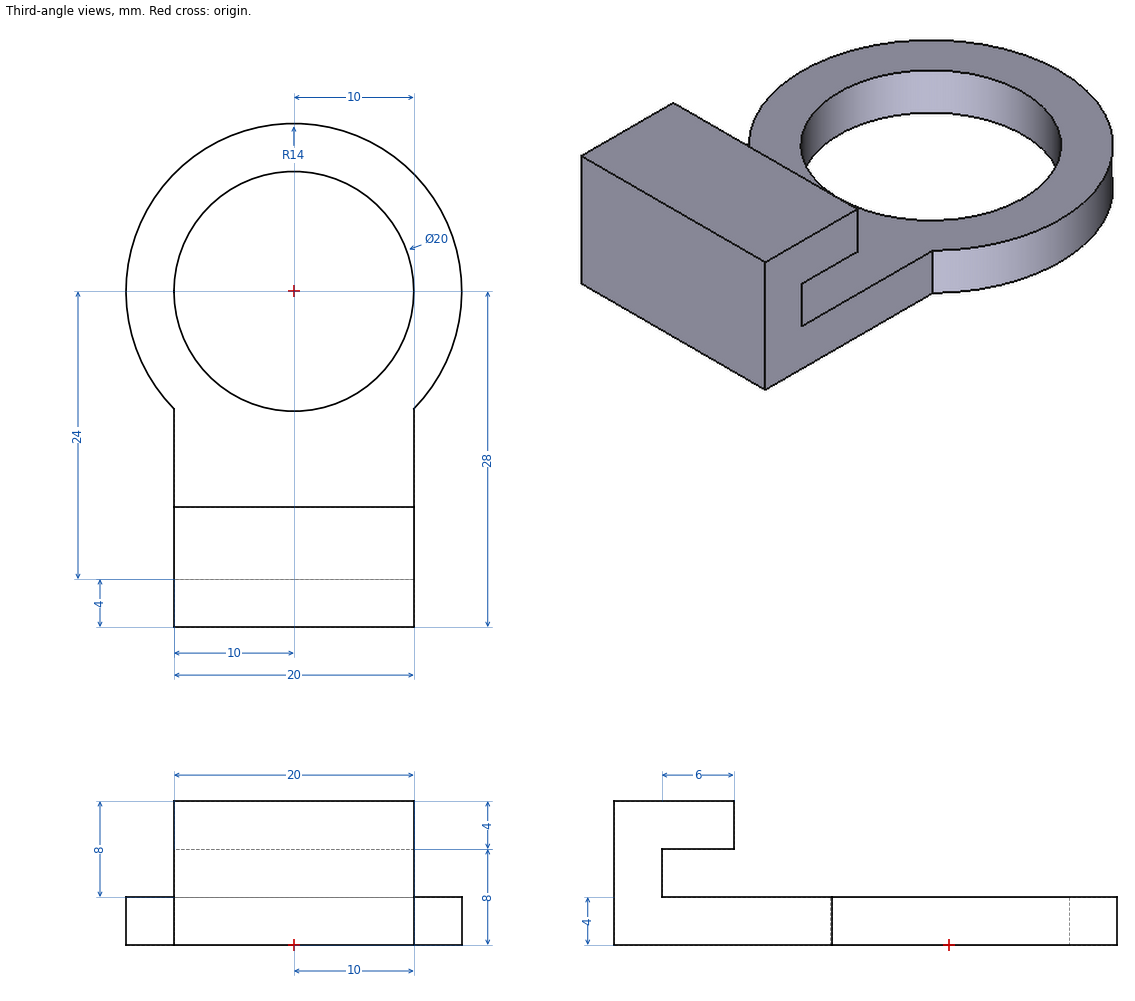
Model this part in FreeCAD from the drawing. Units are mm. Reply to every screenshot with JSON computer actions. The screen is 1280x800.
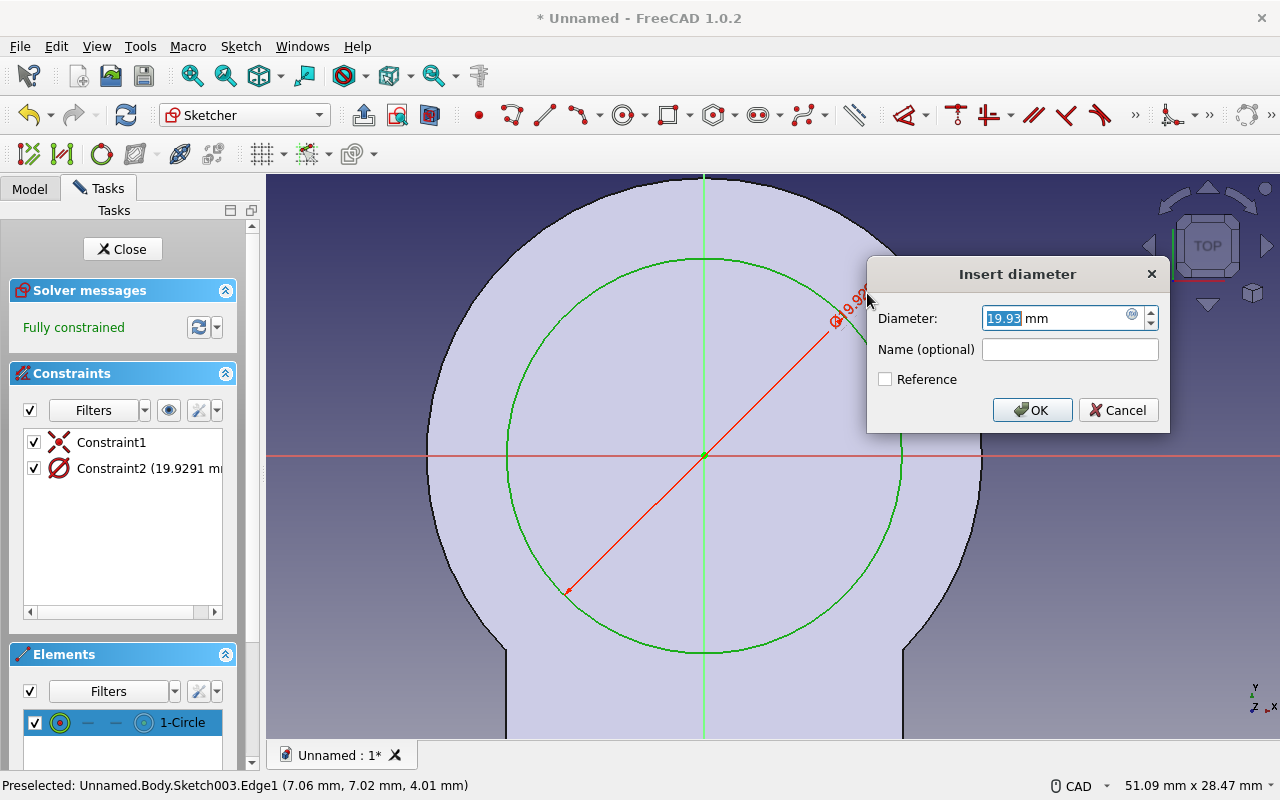
{"action": "type", "text": "20"}
{"action": "key", "text": "Return"}
{"action": "key", "text": "Escape"}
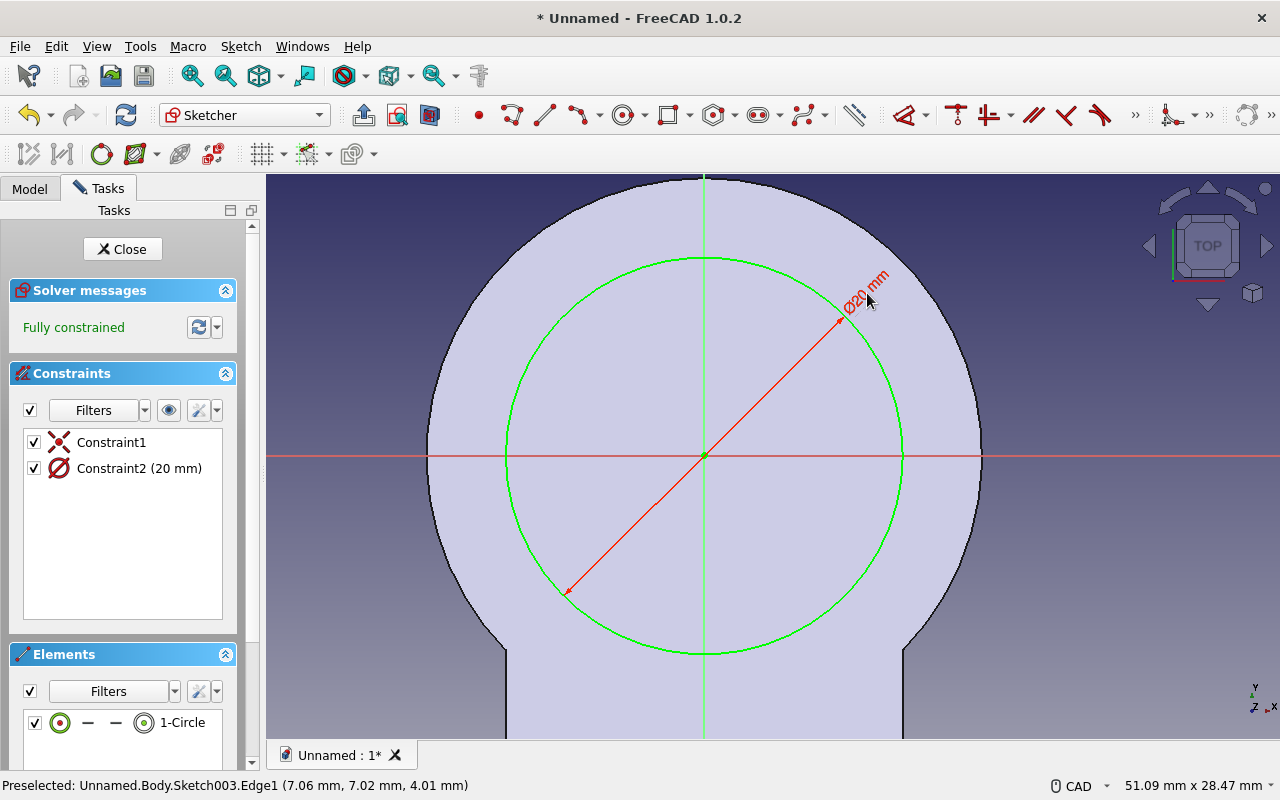
{"action": "left_click", "coordinate": [123, 249]}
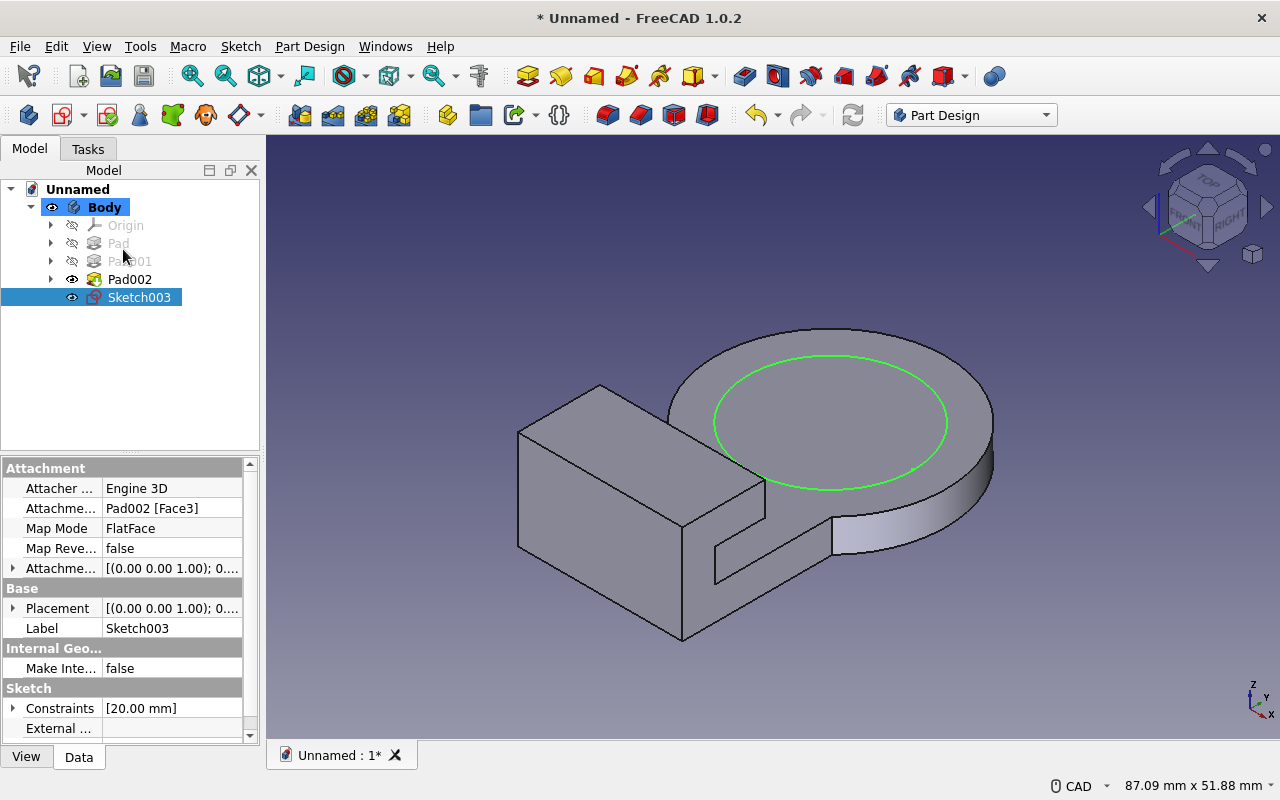
{"action": "left_click", "coordinate": [745, 76]}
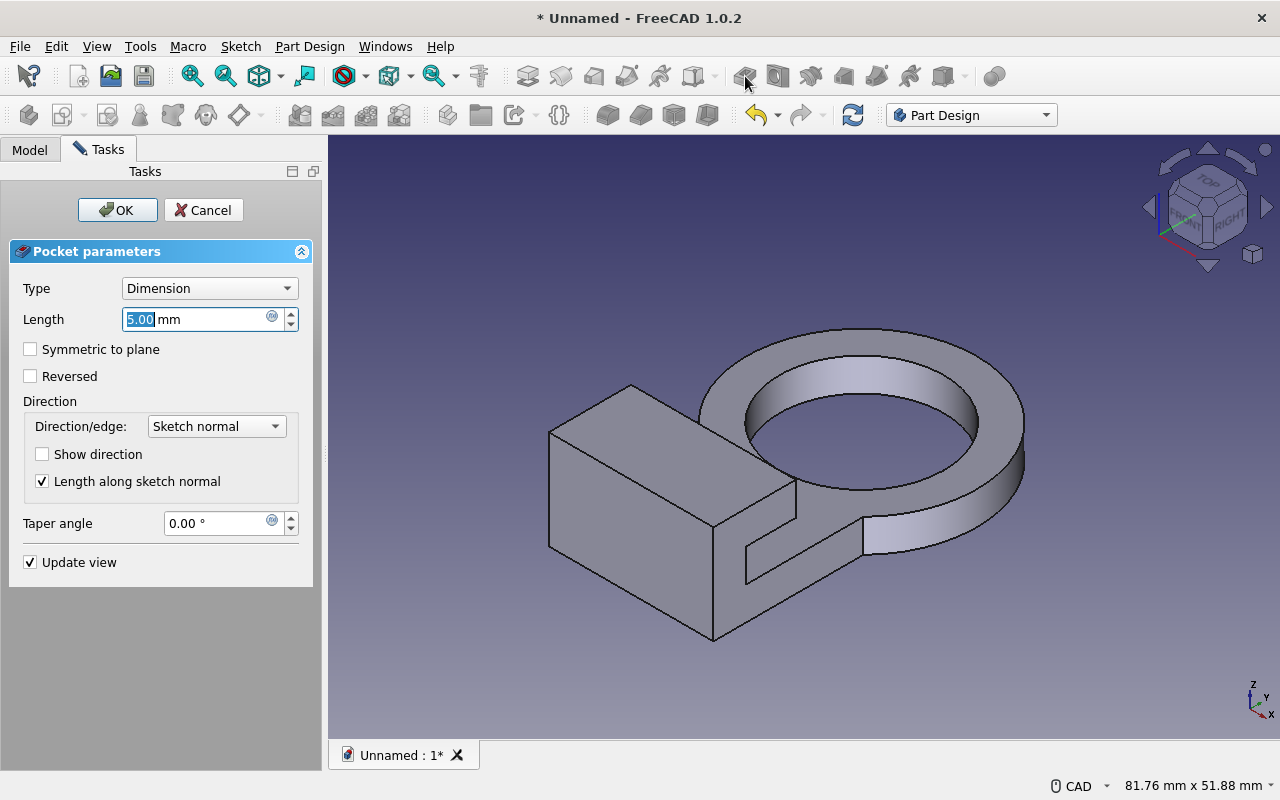
{"action": "left_click", "coordinate": [210, 288]}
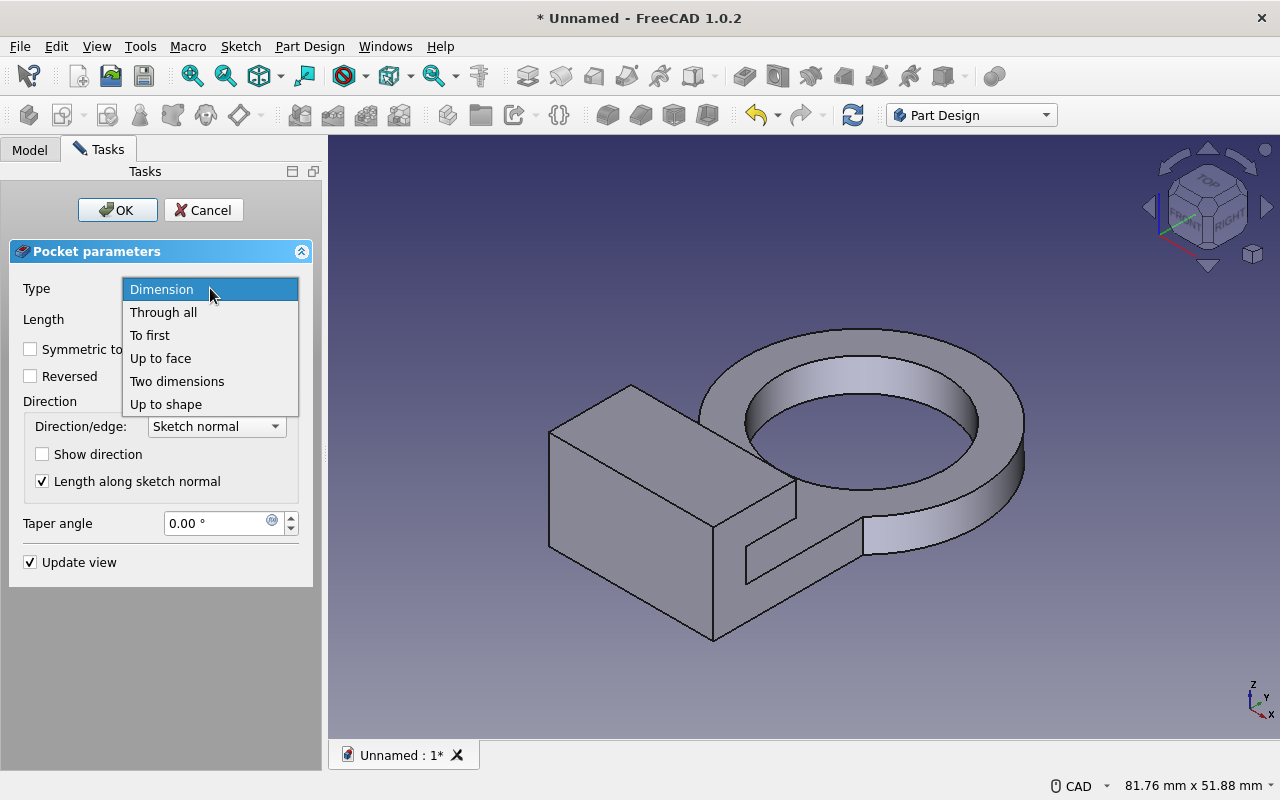
{"action": "left_click", "coordinate": [208, 312]}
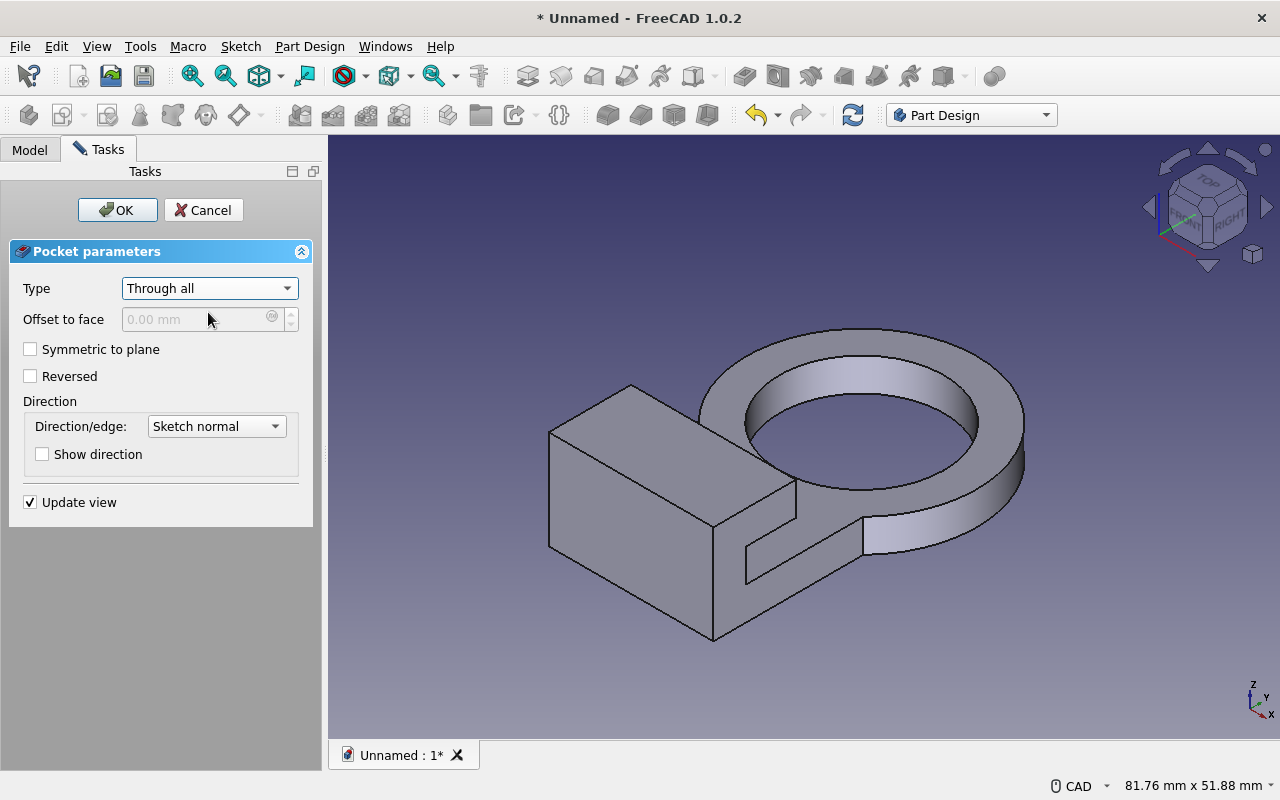
{"action": "left_click", "coordinate": [118, 210]}